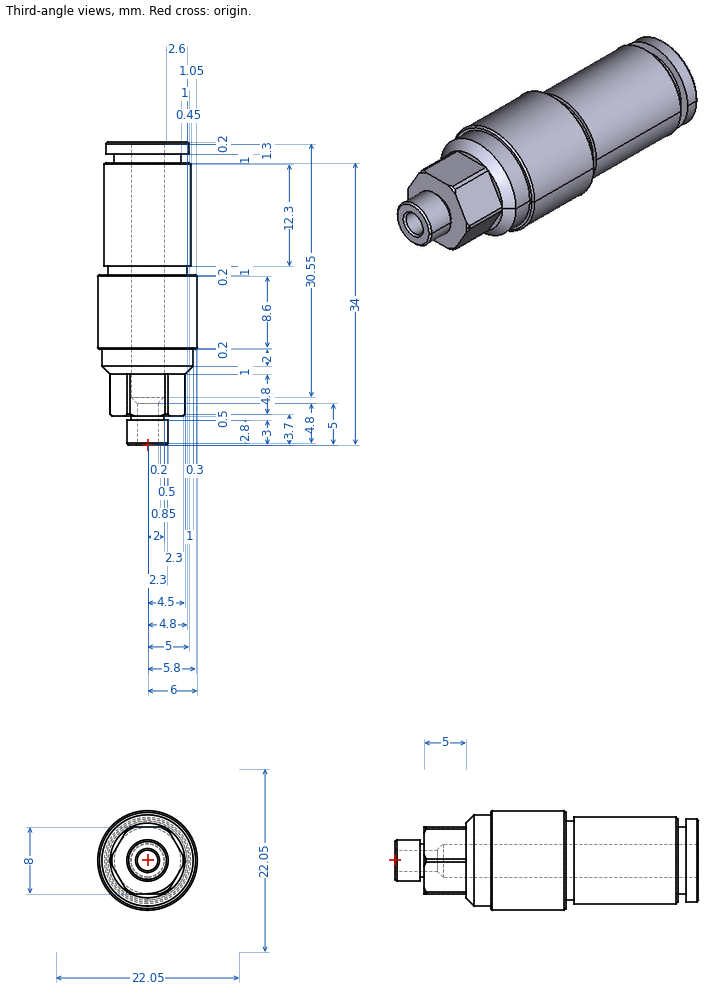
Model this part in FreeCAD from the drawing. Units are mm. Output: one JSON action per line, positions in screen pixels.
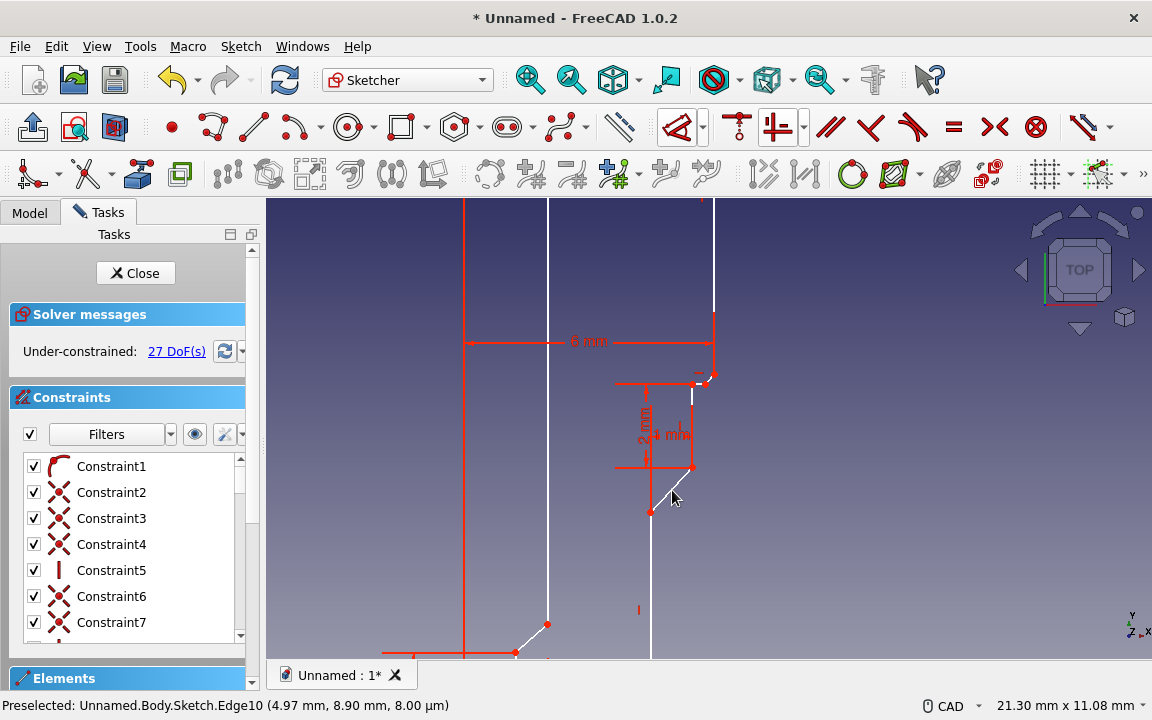
{"action": "left_click", "coordinate": [663, 499]}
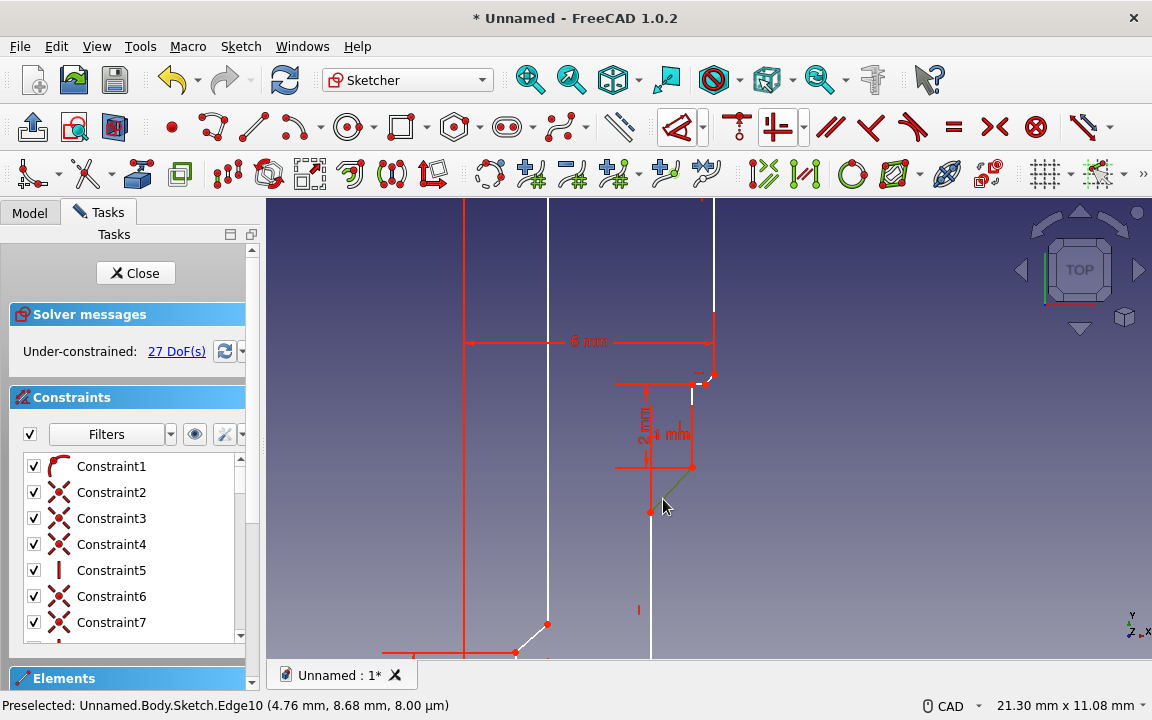
{"action": "left_click", "coordinate": [702, 128]}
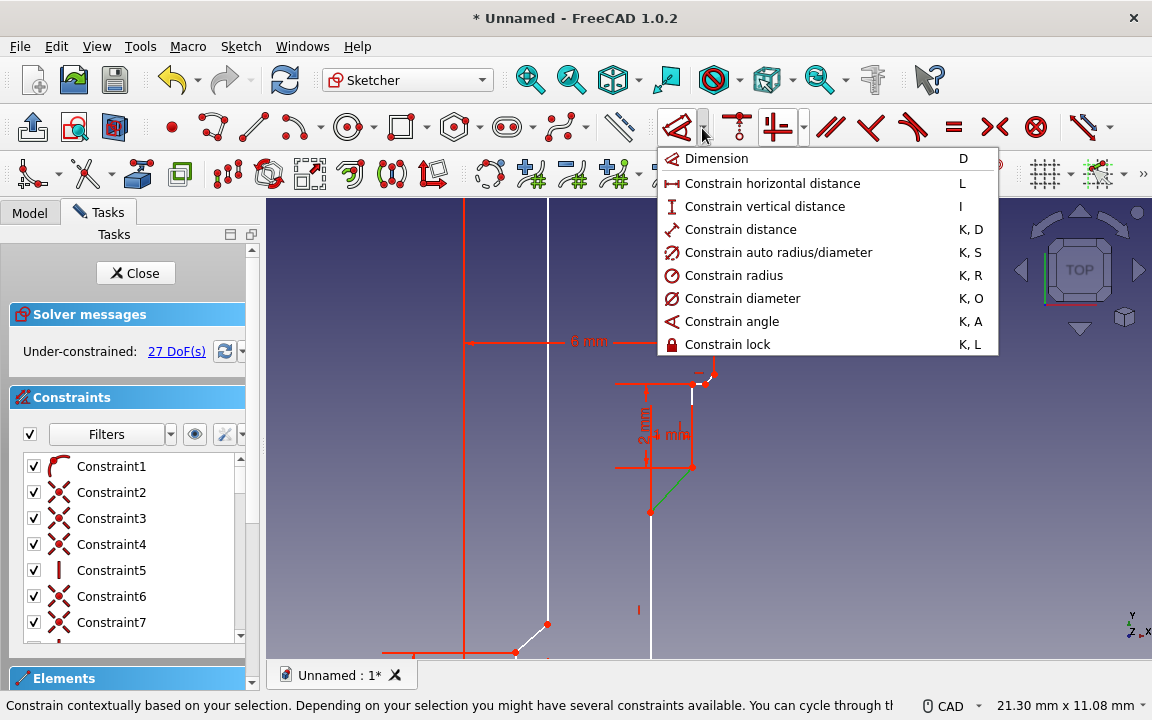
{"action": "left_click", "coordinate": [828, 206]}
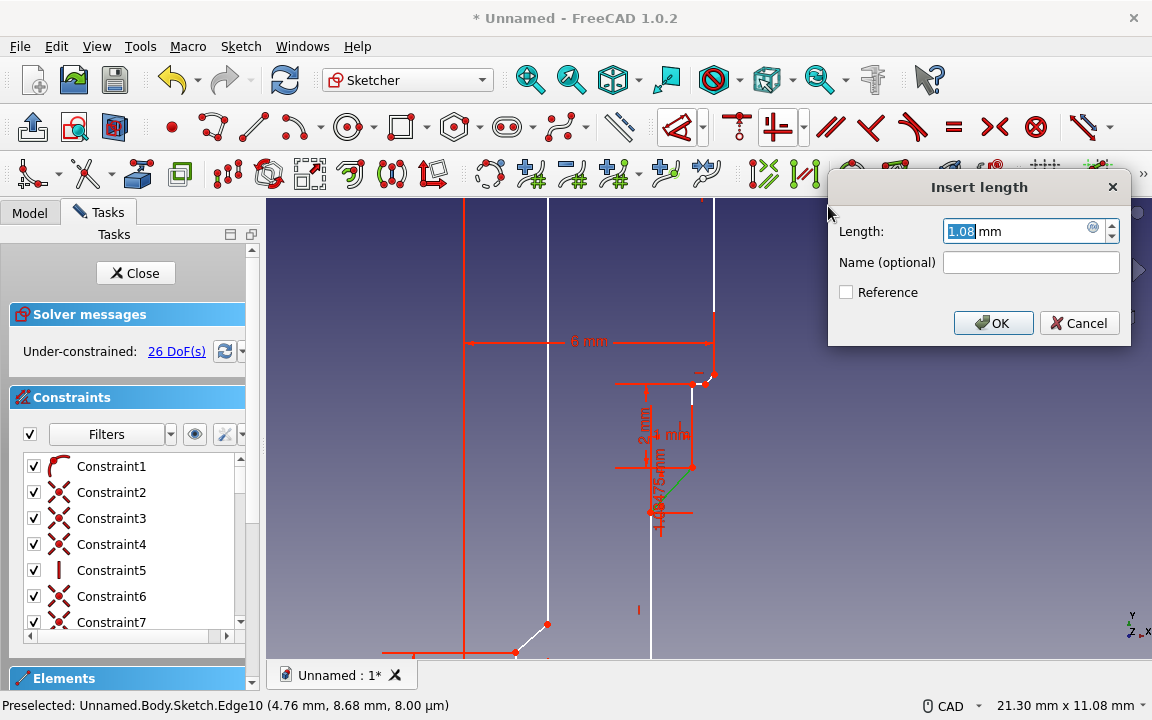
{"action": "type", "text": "1"}
{"action": "key", "text": "Return"}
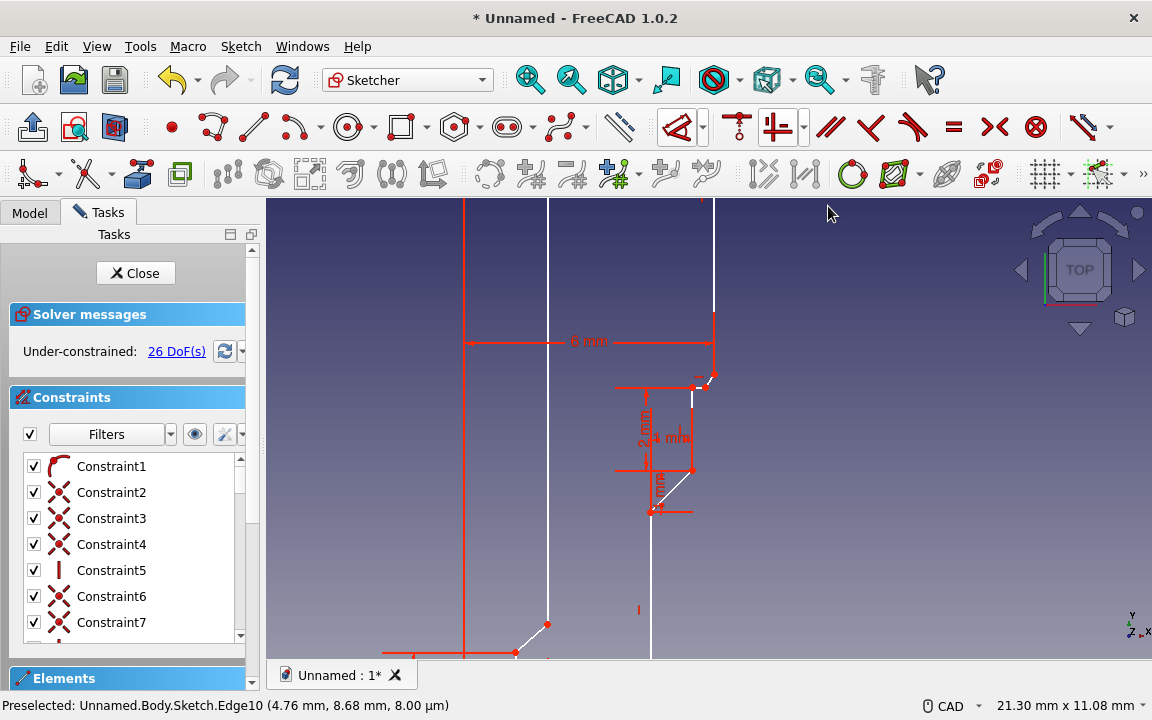
{"action": "scroll", "coordinate": [653, 511], "scroll_direction": "down", "scroll_amount": 8}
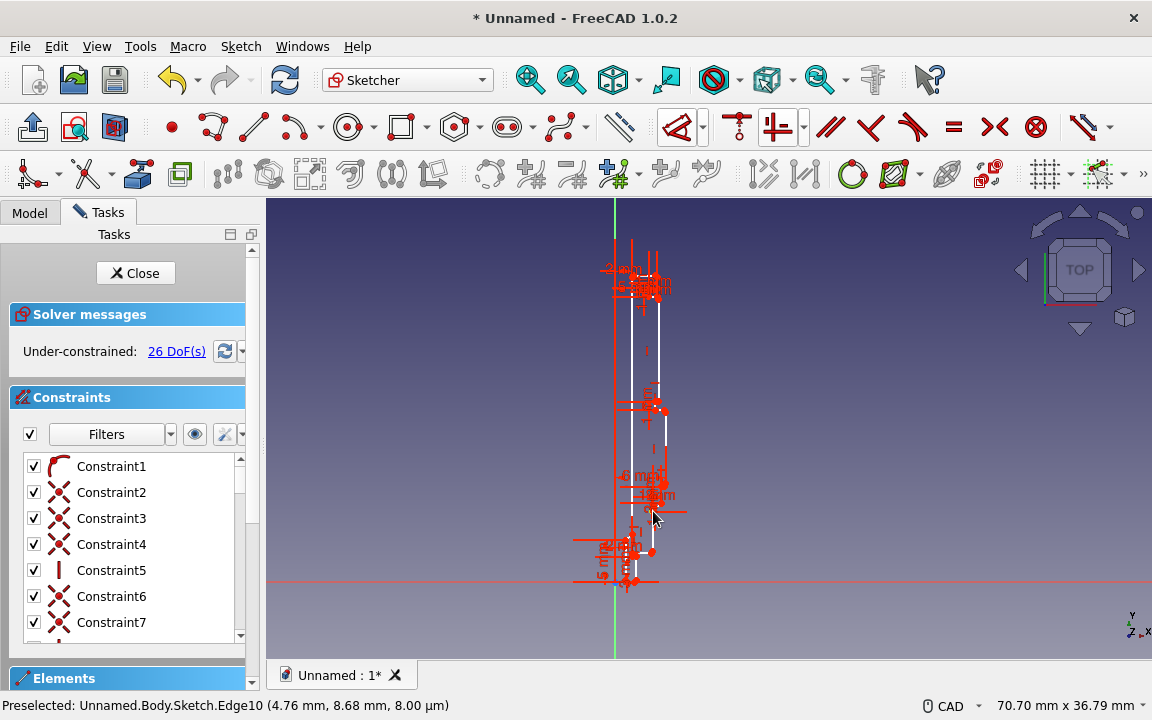
{"action": "scroll", "coordinate": [636, 573], "scroll_direction": "up", "scroll_amount": 4}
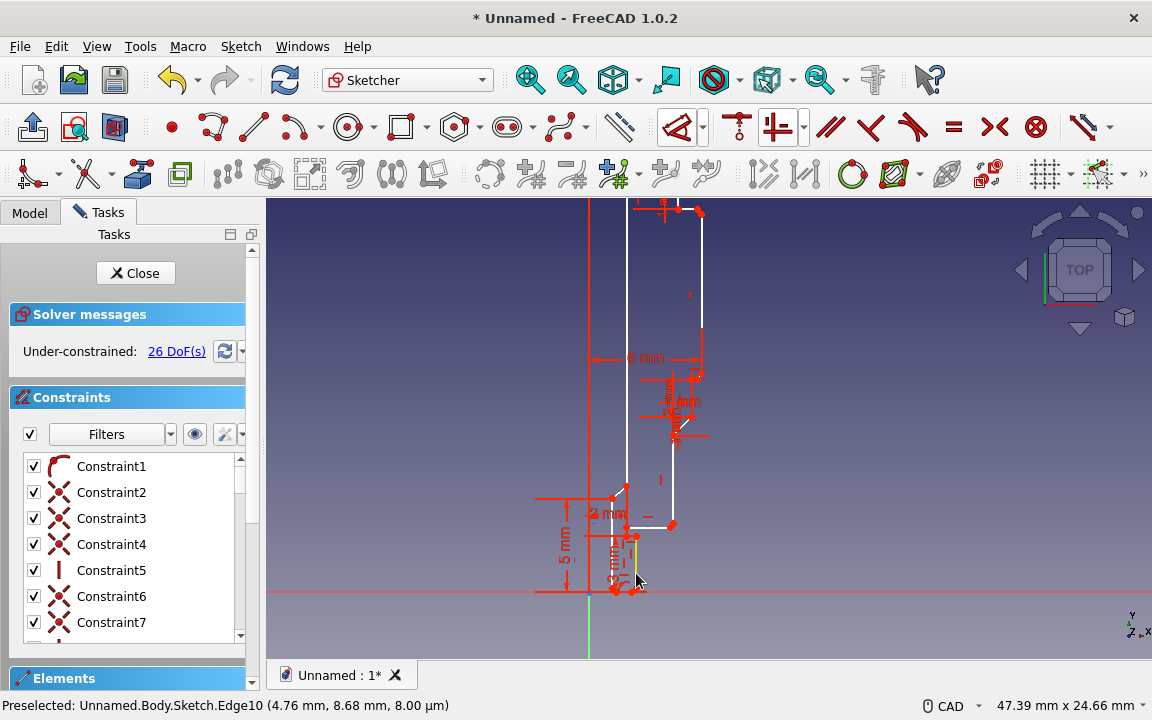
{"action": "left_click", "coordinate": [636, 573]}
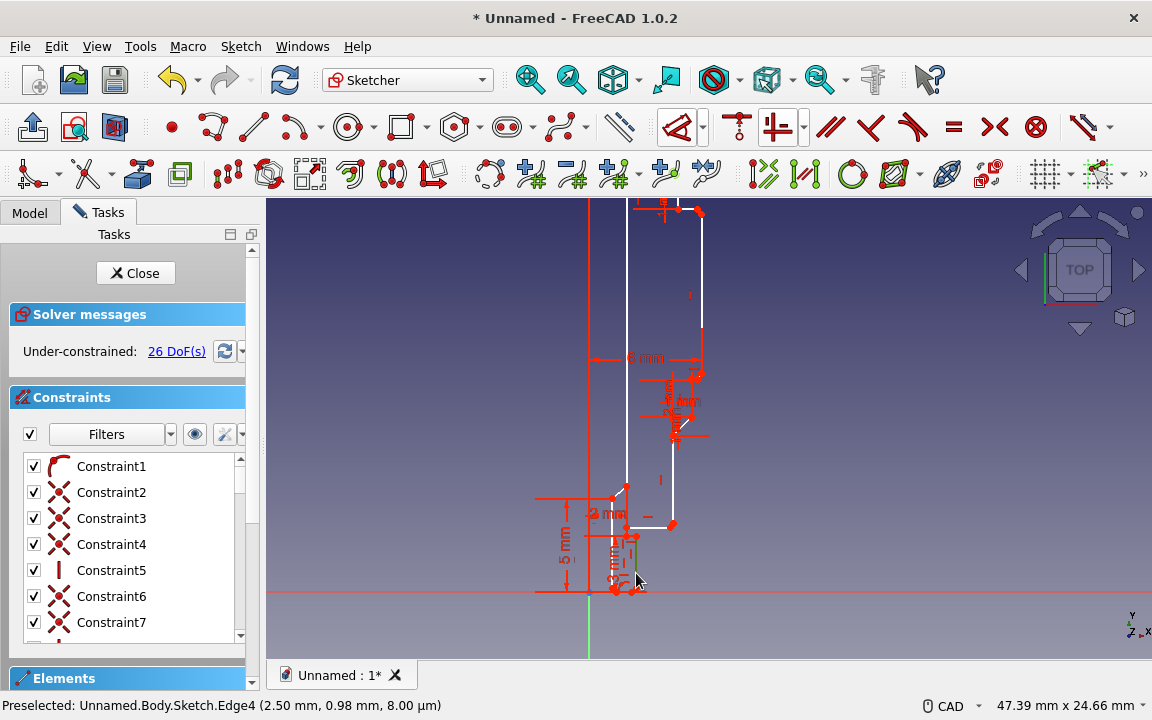
{"action": "key", "text": "i"}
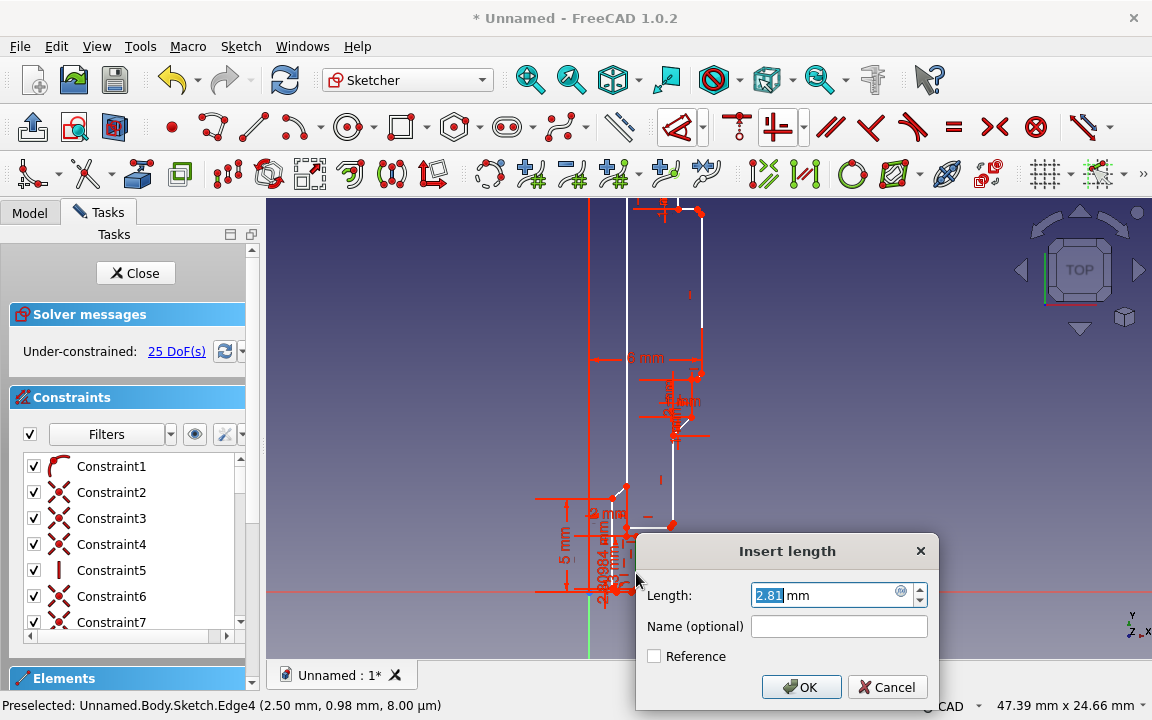
{"action": "type", "text": "2.8"}
{"action": "key", "text": "Return"}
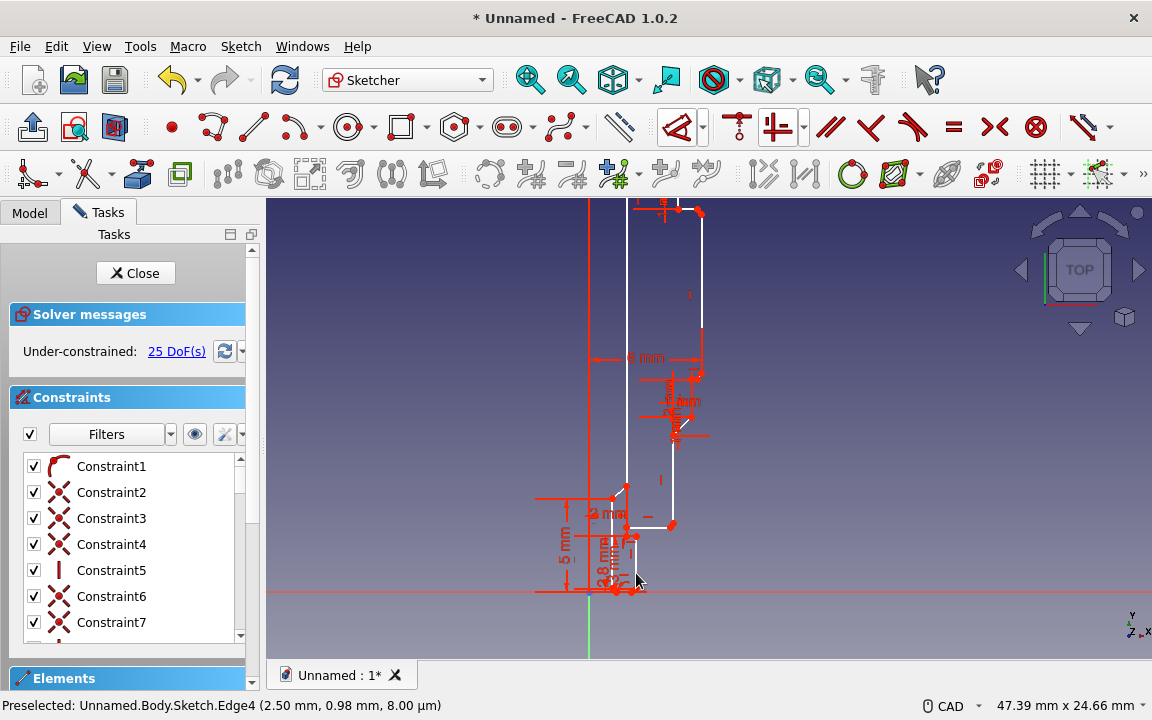
{"action": "scroll", "coordinate": [631, 536], "scroll_direction": "up", "scroll_amount": 8}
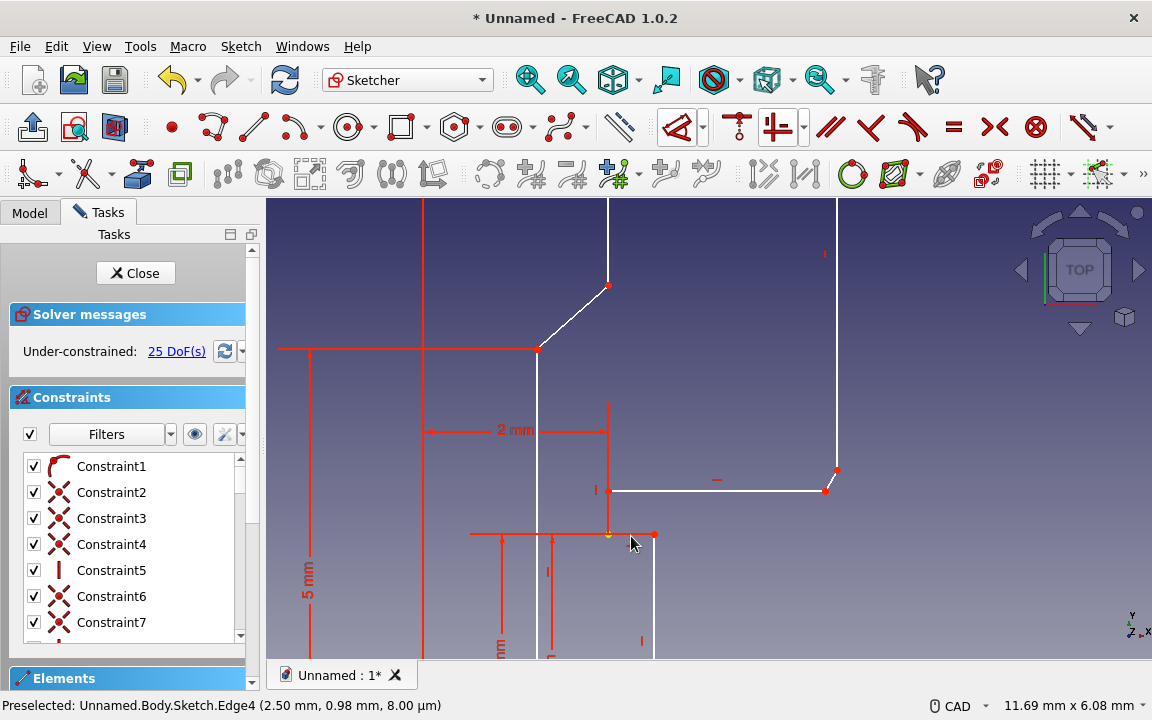
{"action": "left_click", "coordinate": [631, 534]}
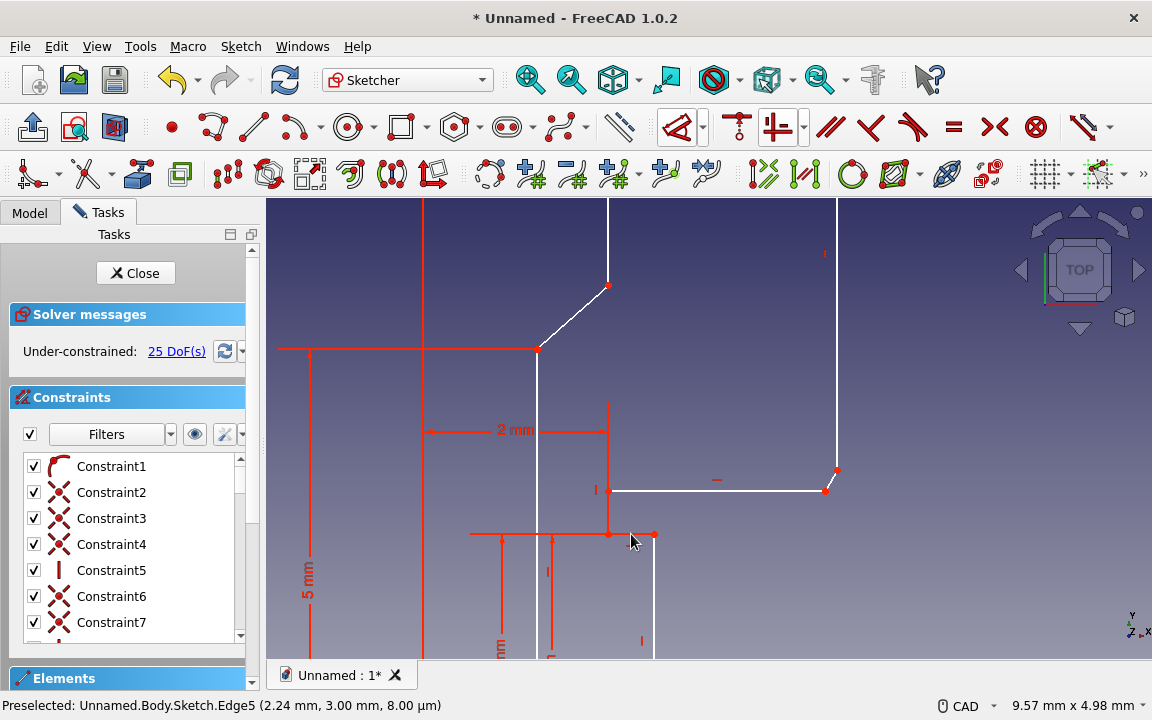
{"action": "key", "text": "l"}